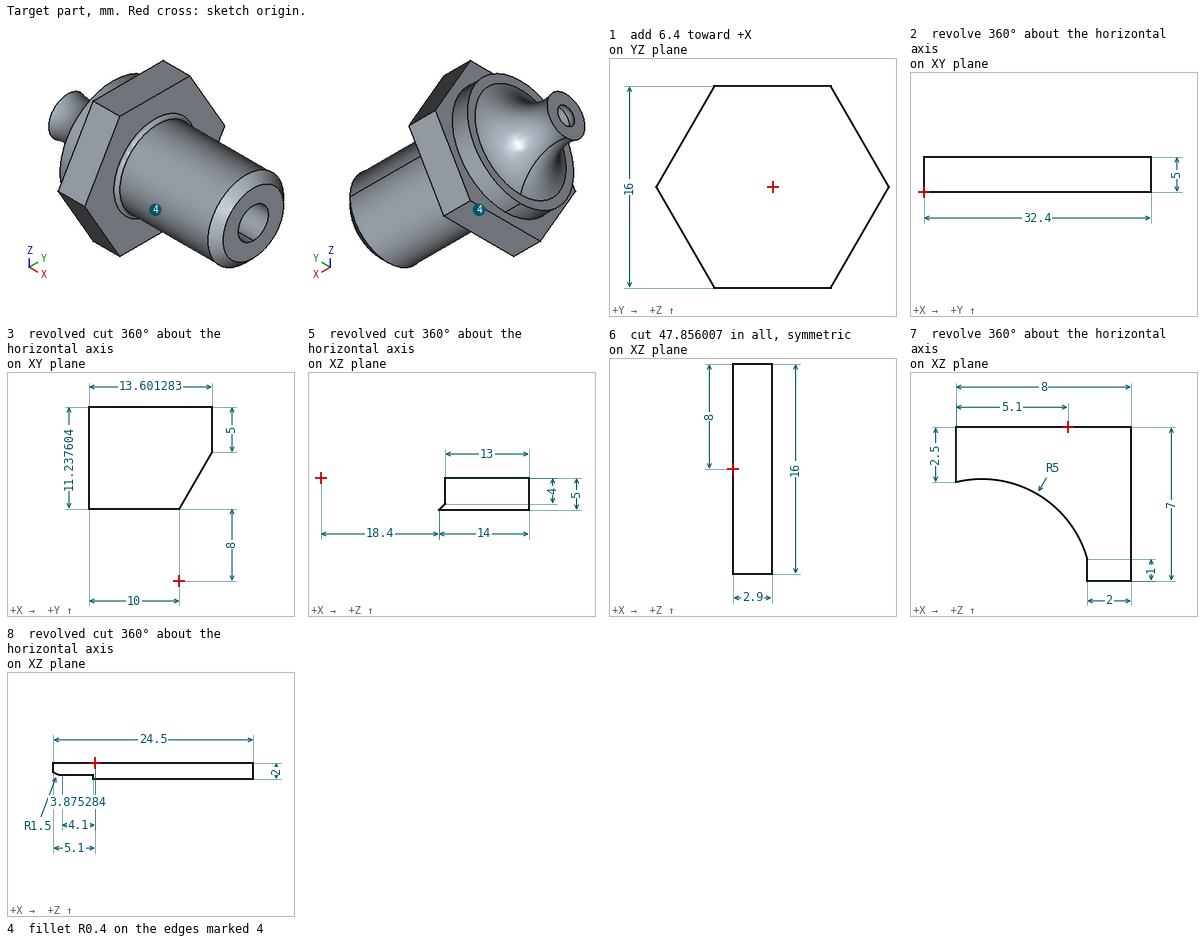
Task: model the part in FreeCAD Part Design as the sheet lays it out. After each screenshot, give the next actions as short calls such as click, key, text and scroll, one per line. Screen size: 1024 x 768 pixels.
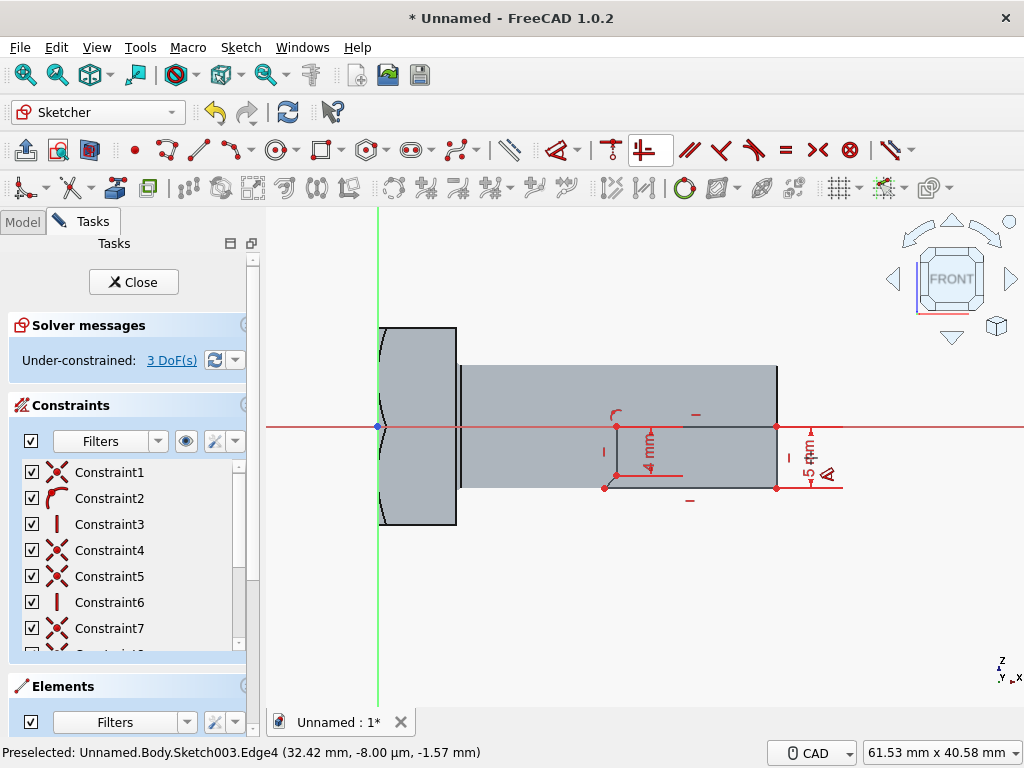
click(665, 427)
click(697, 393)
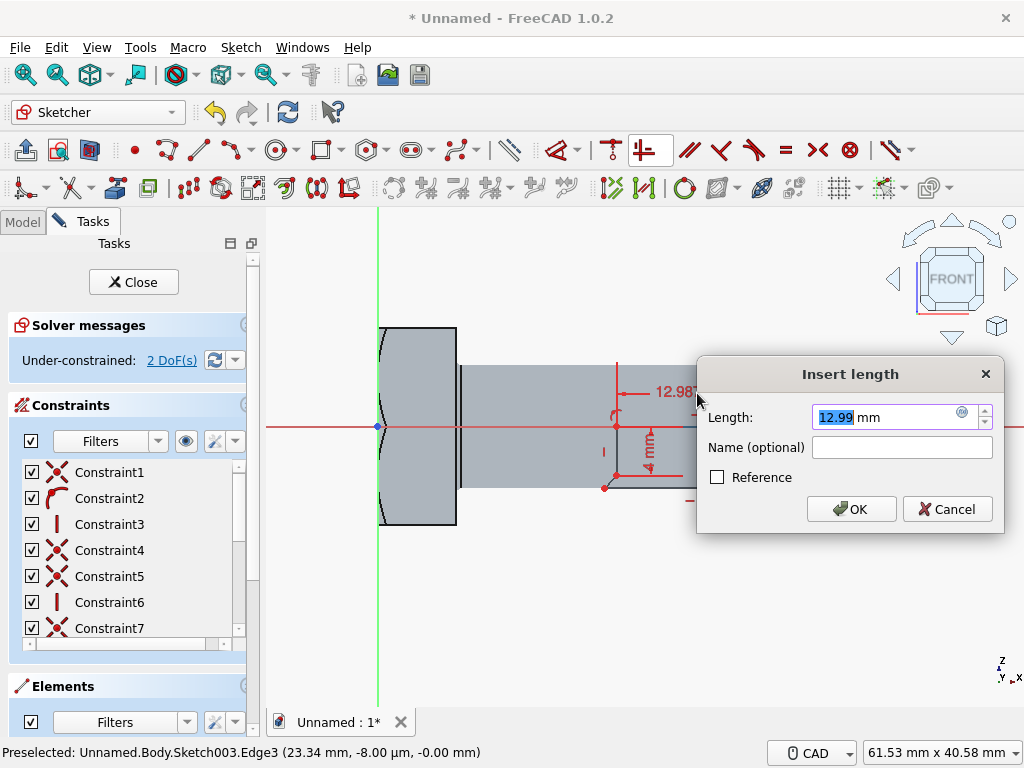
text(13)
key(Return)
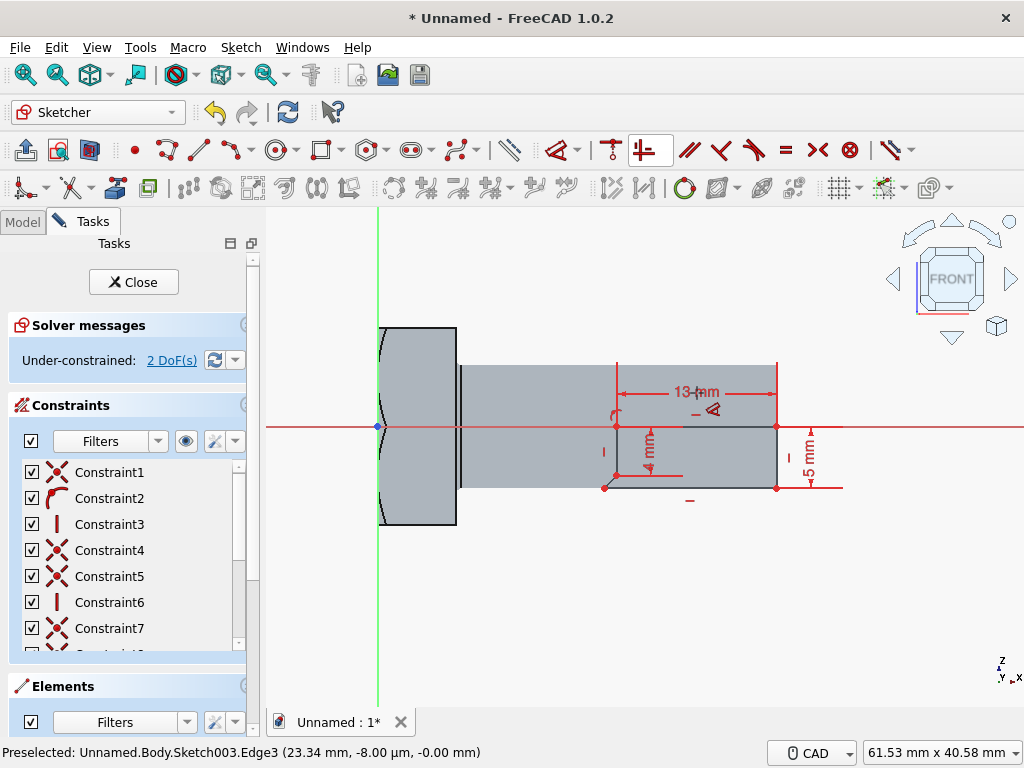
click(725, 488)
click(691, 522)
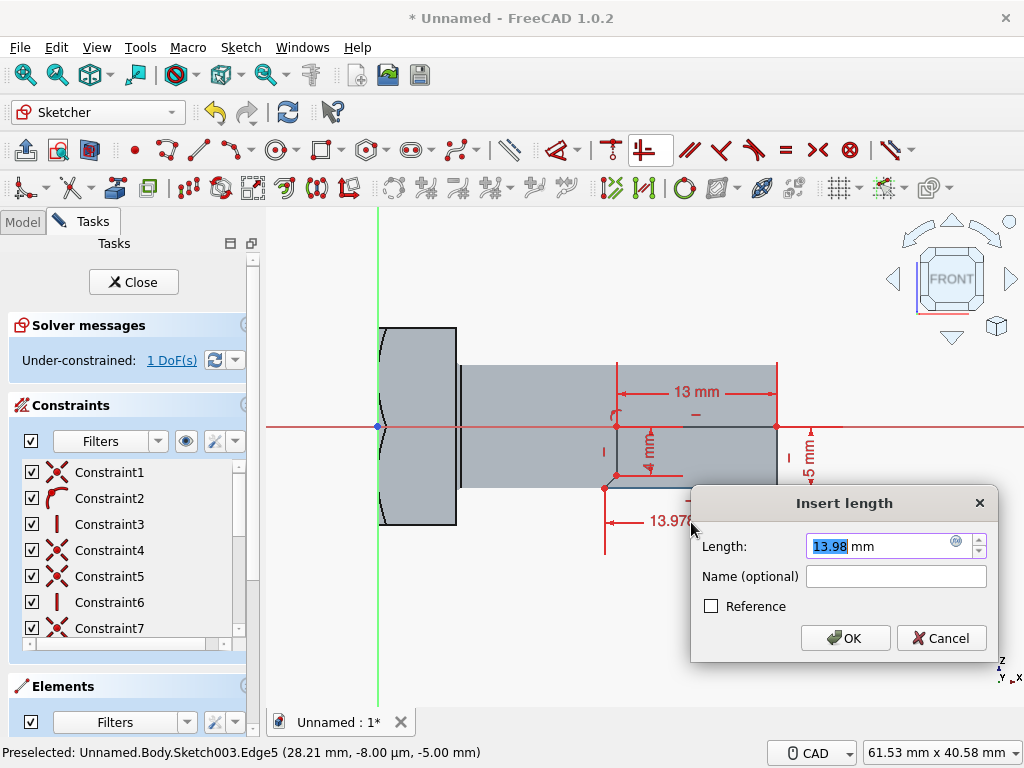
text(14)
key(Return)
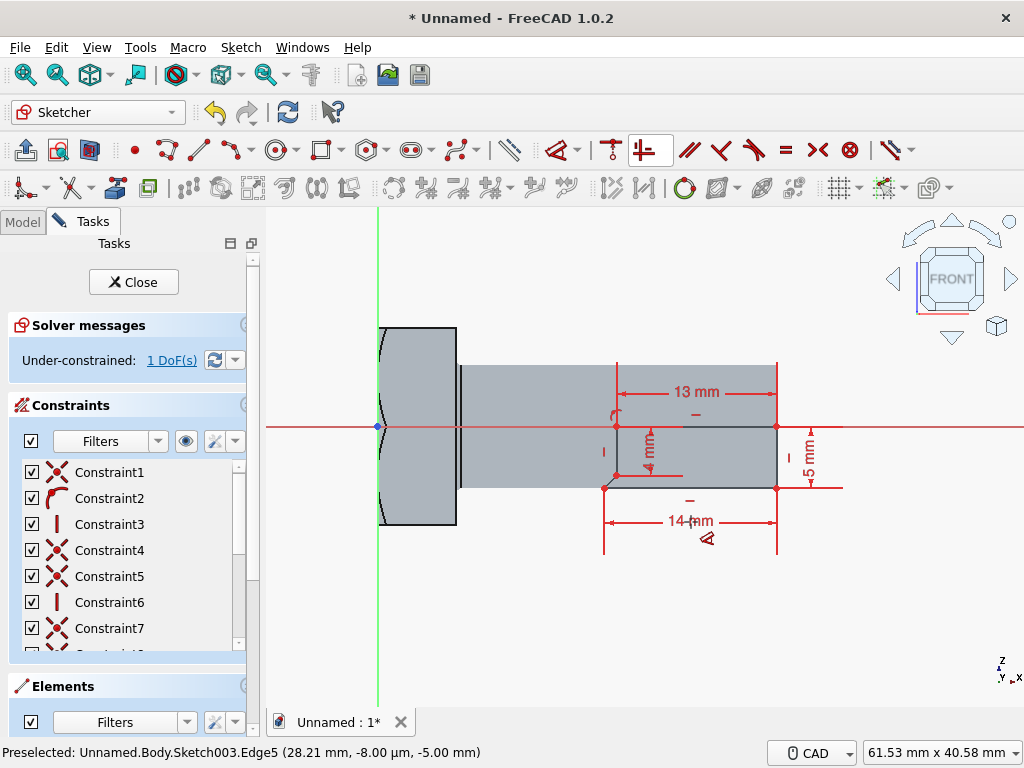
click(604, 488)
click(491, 522)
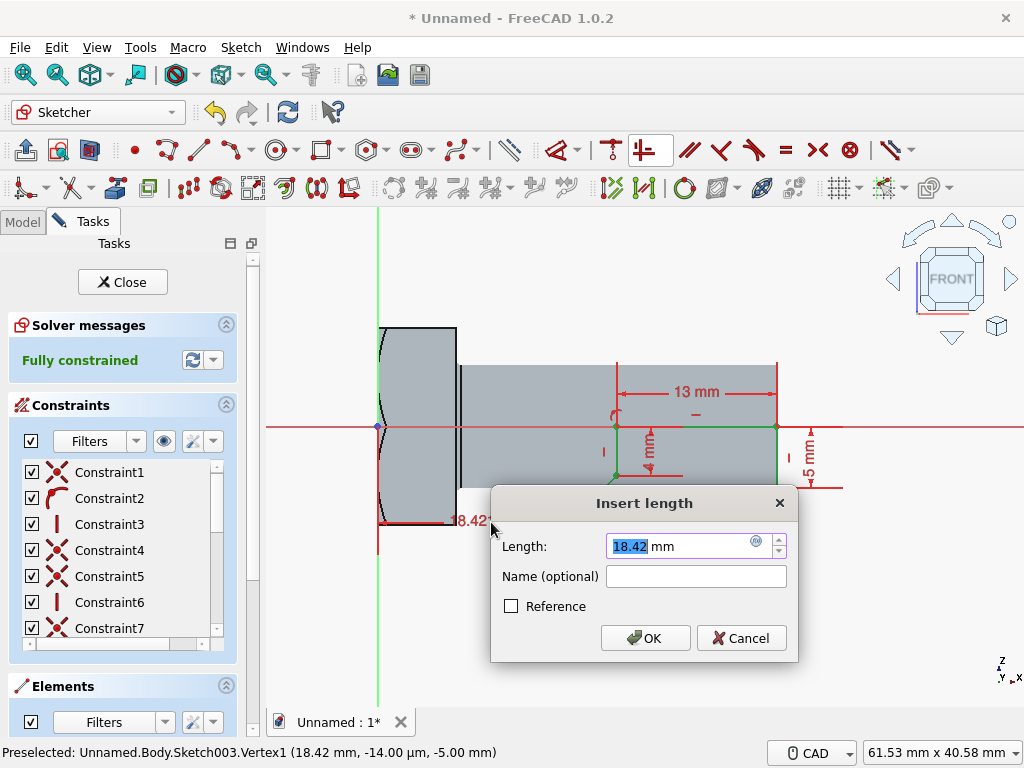
text(18.4)
key(Return)
key(Escape)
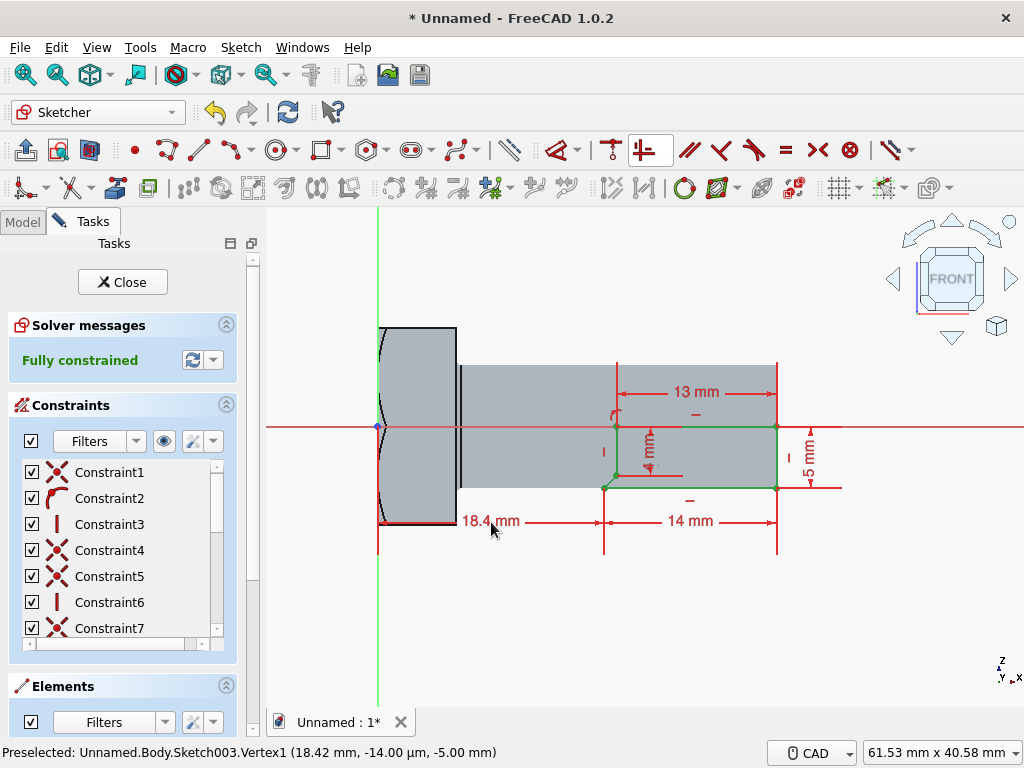
click(123, 282)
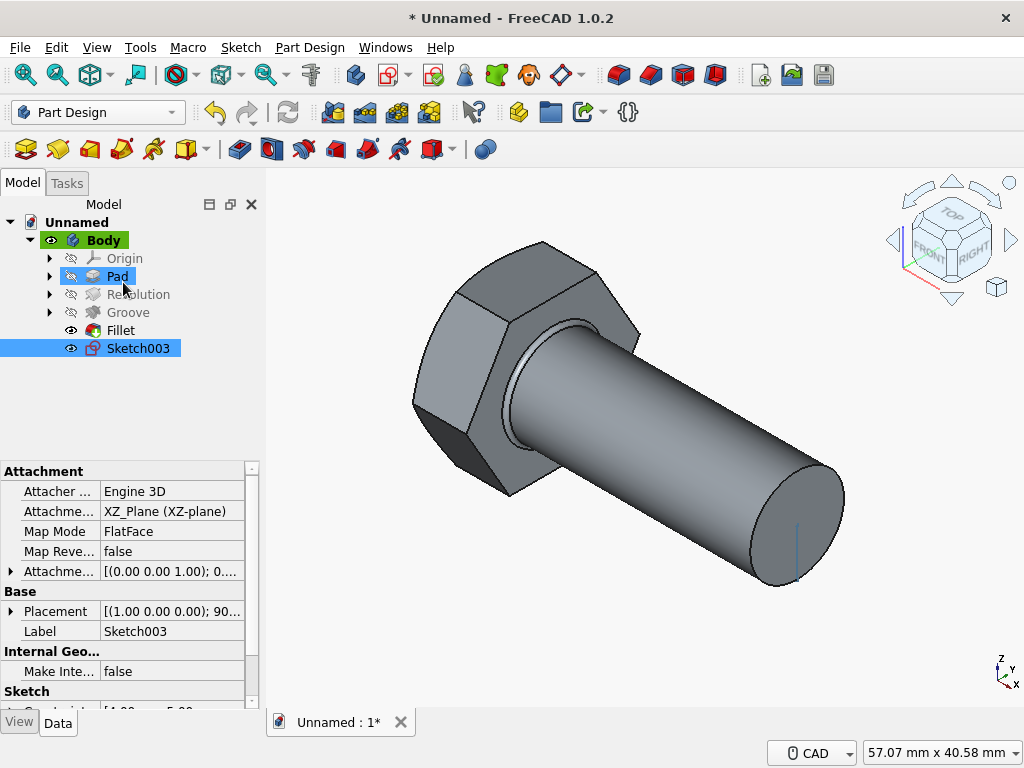
click(304, 150)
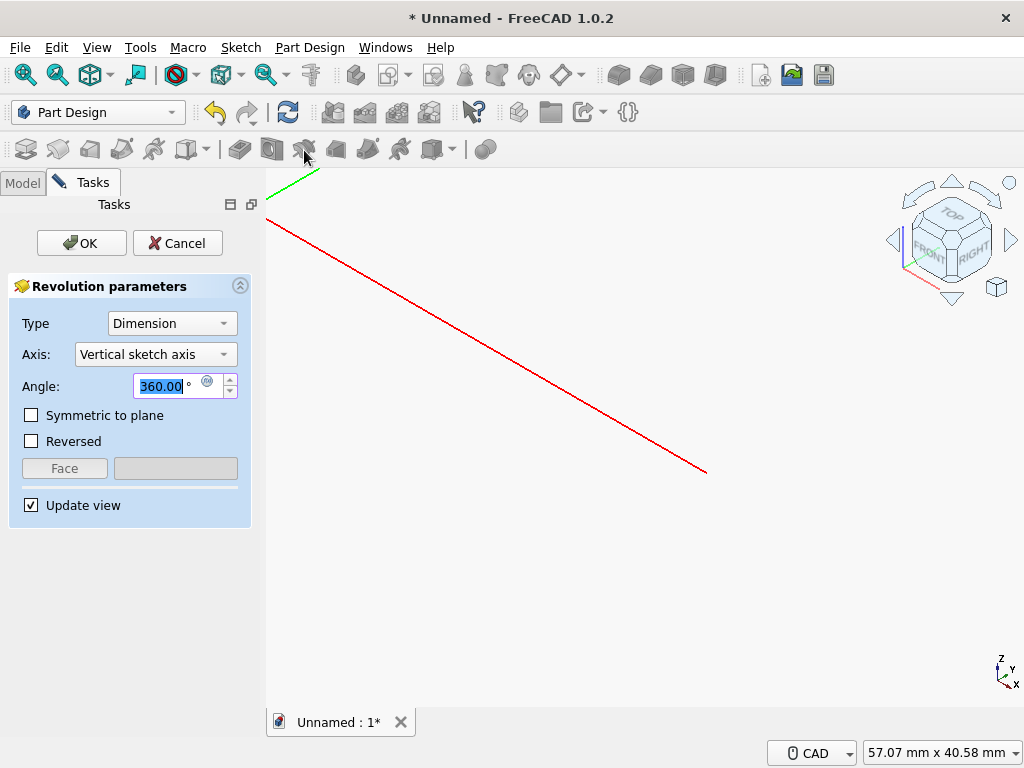
click(156, 354)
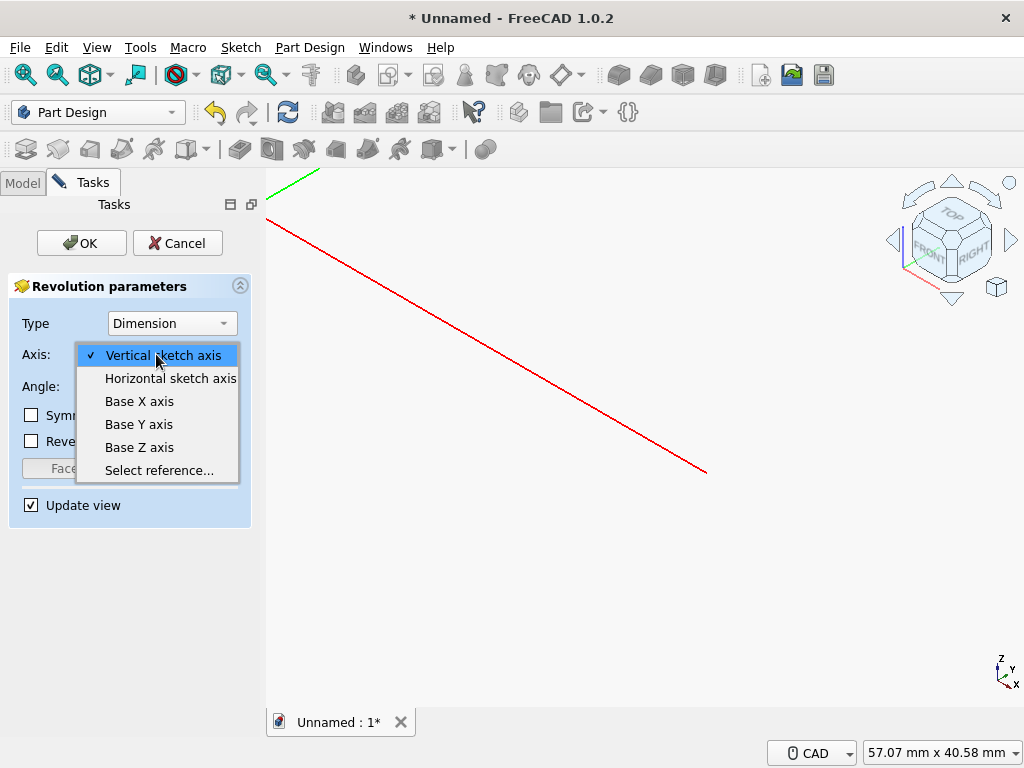
click(156, 378)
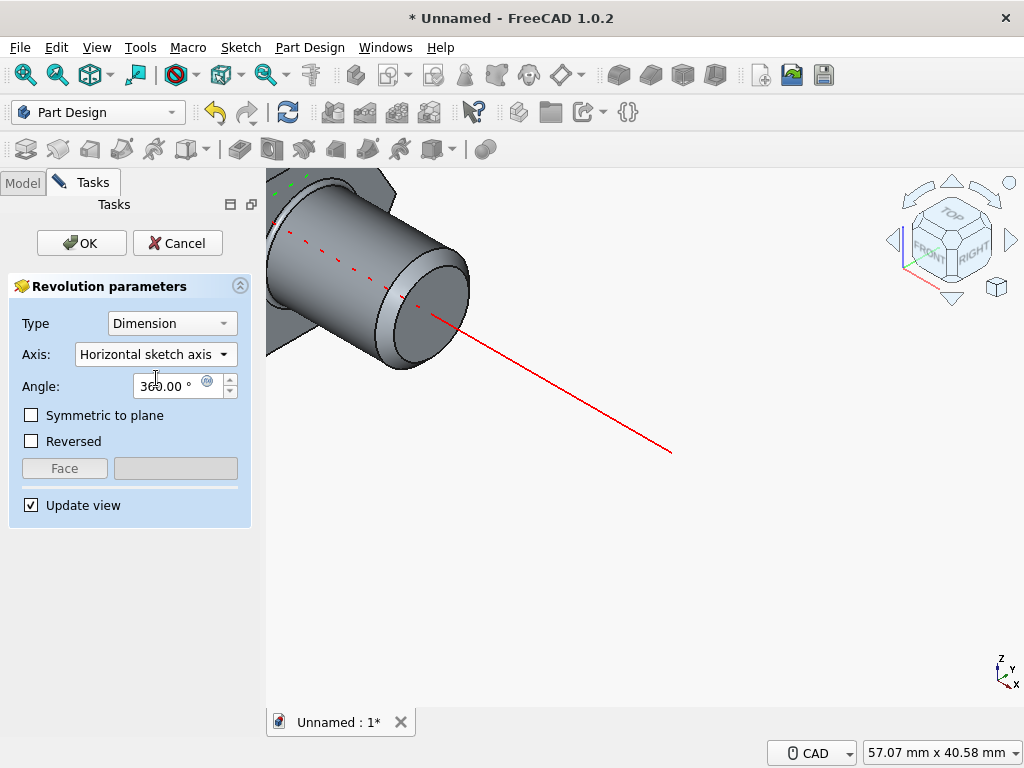
click(82, 243)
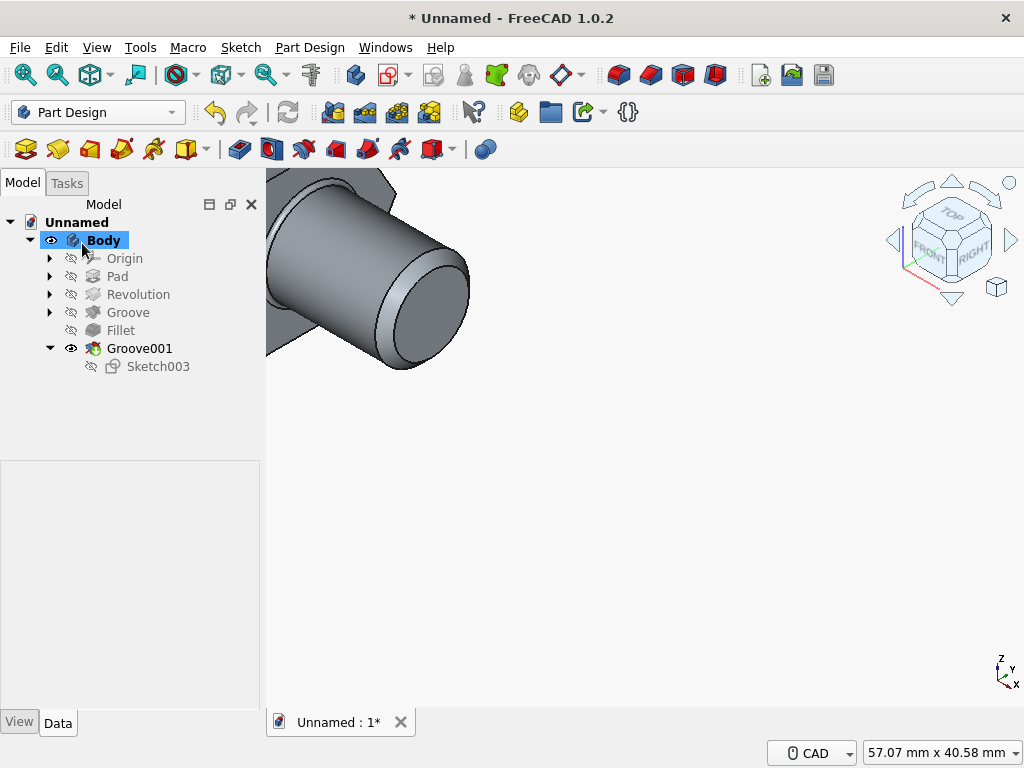
click(26, 76)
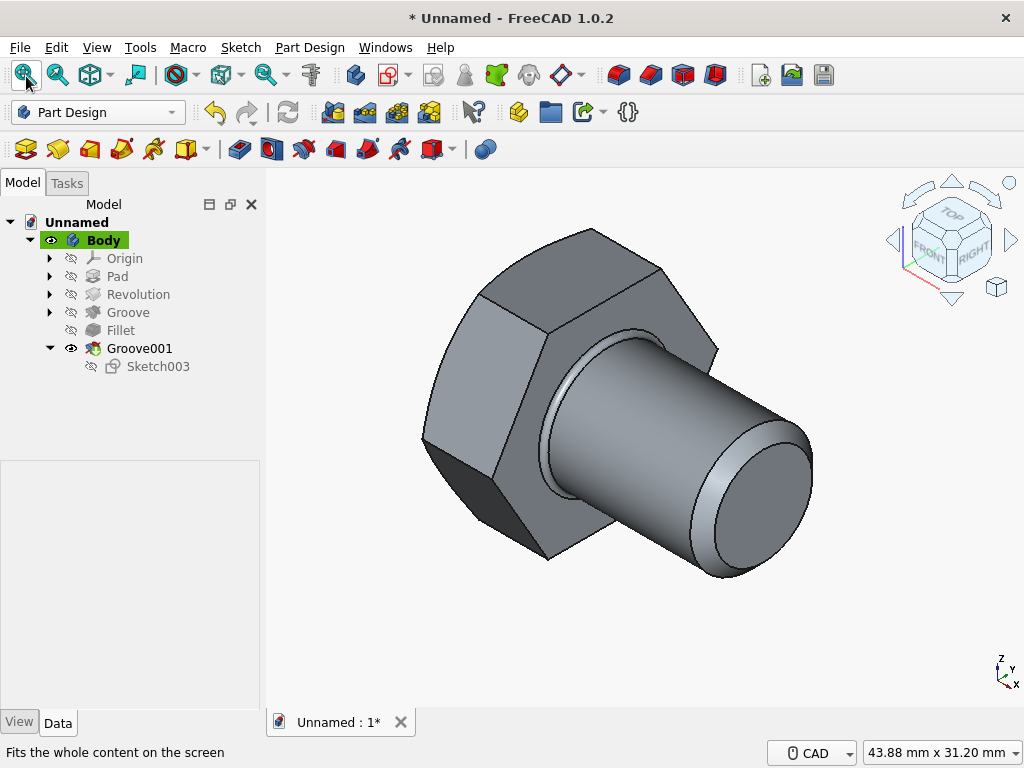
click(388, 76)